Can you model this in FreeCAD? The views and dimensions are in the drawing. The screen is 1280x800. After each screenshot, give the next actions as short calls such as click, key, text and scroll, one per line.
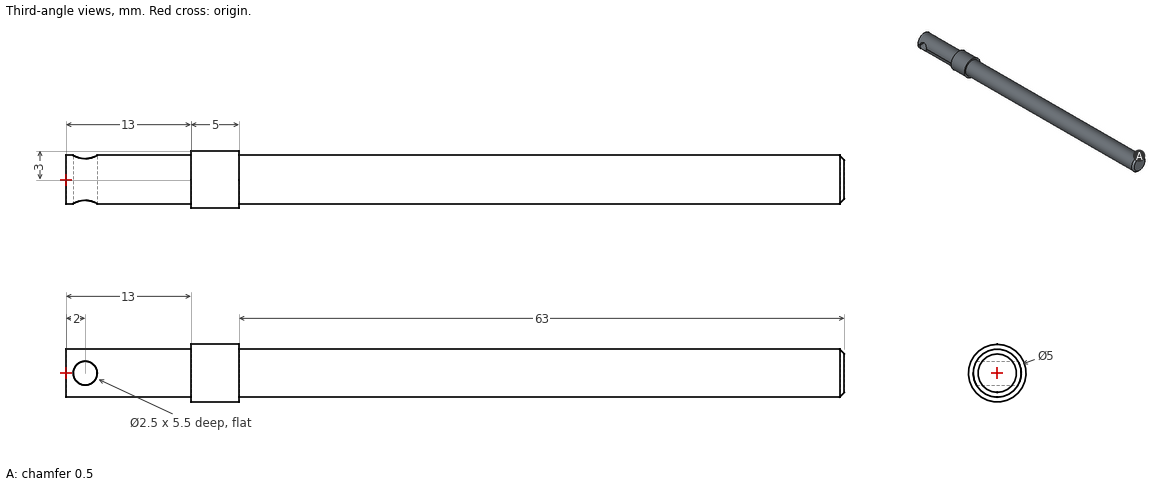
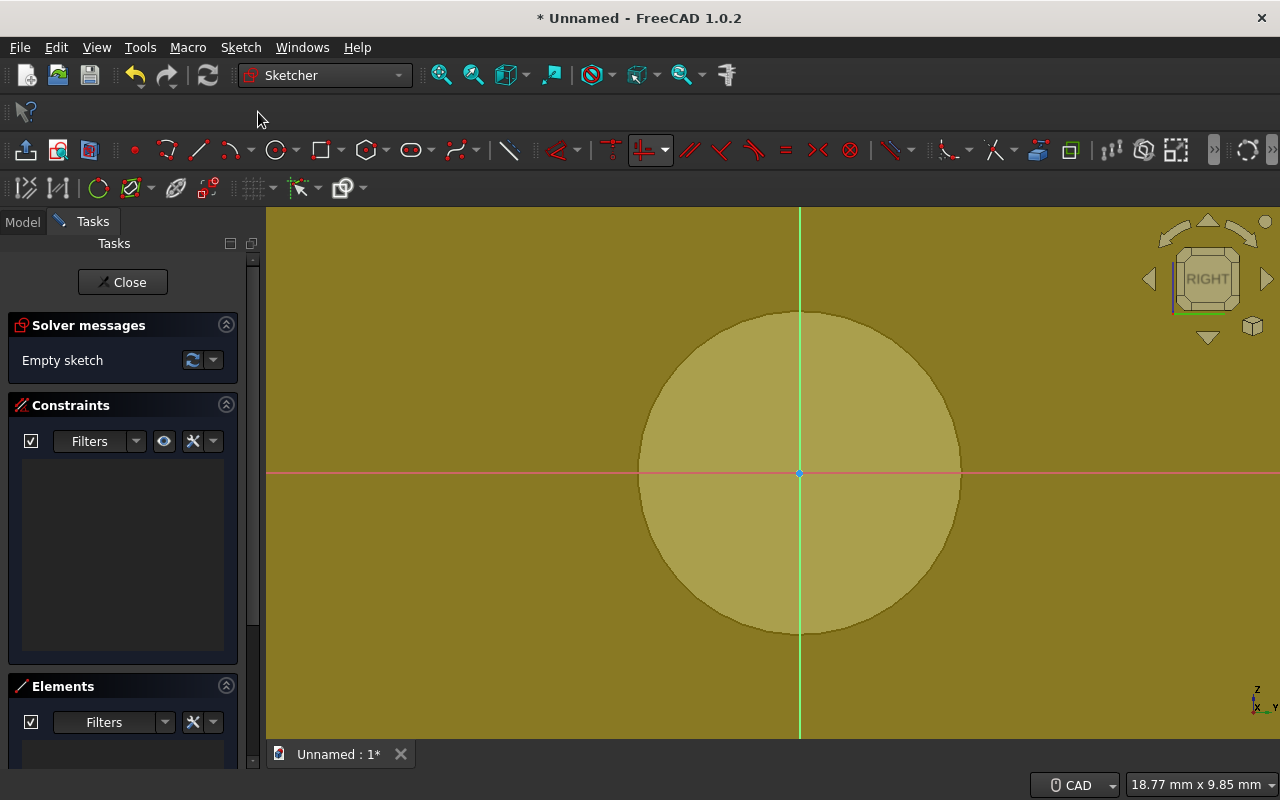
click(276, 150)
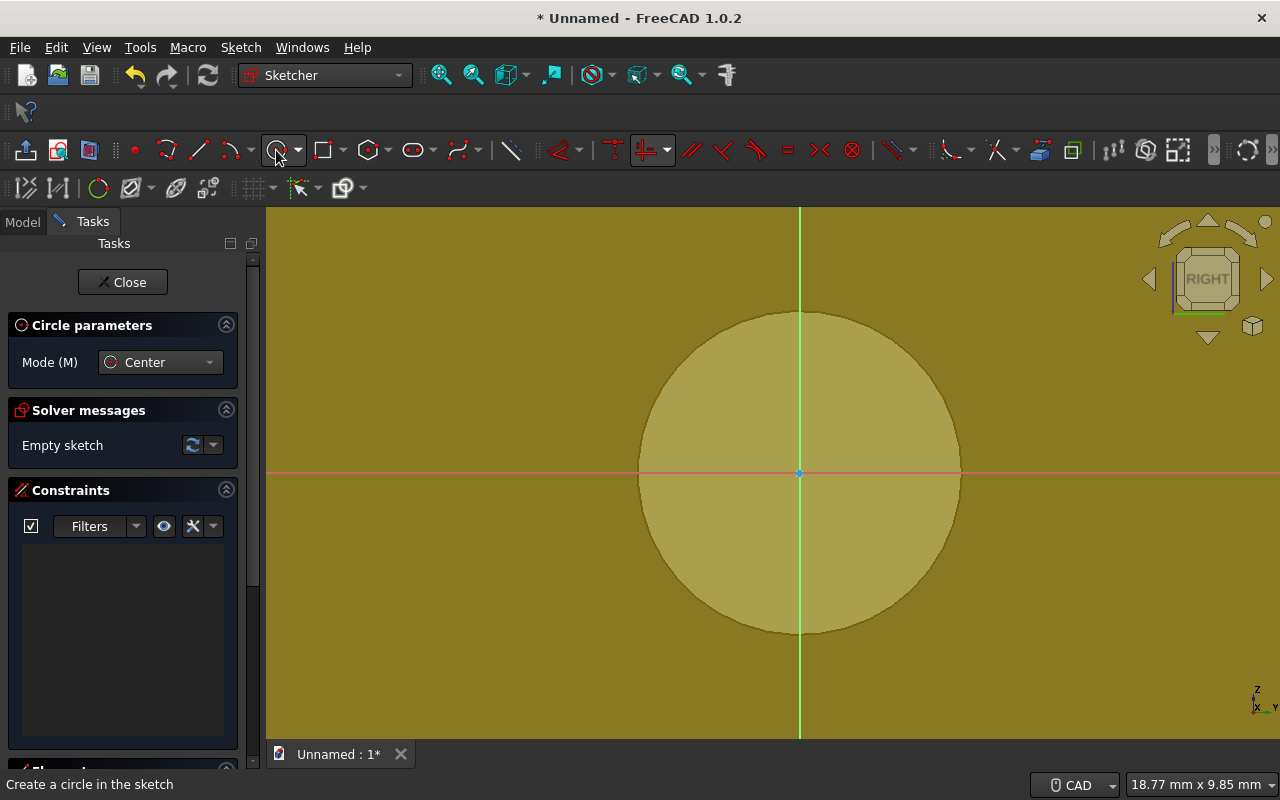
click(800, 473)
move(895, 378)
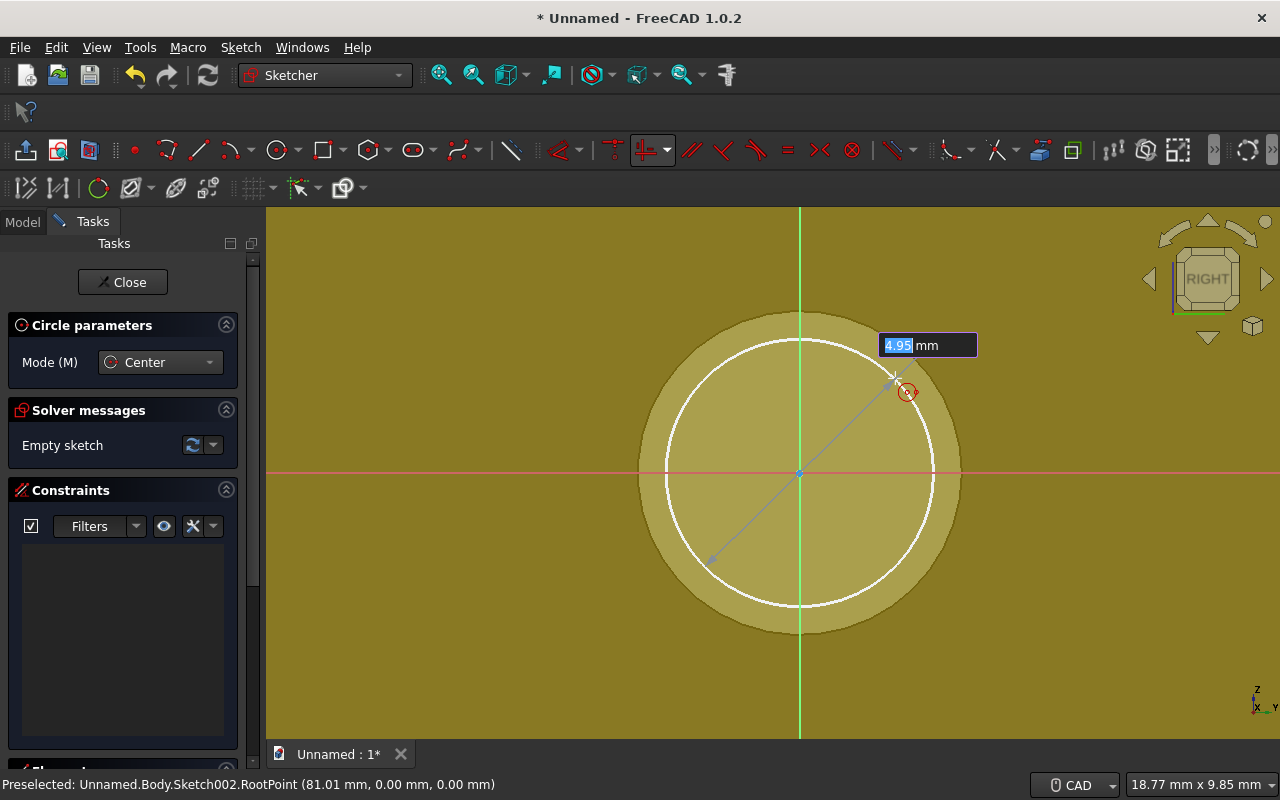
text(5)
key(Return)
key(Escape)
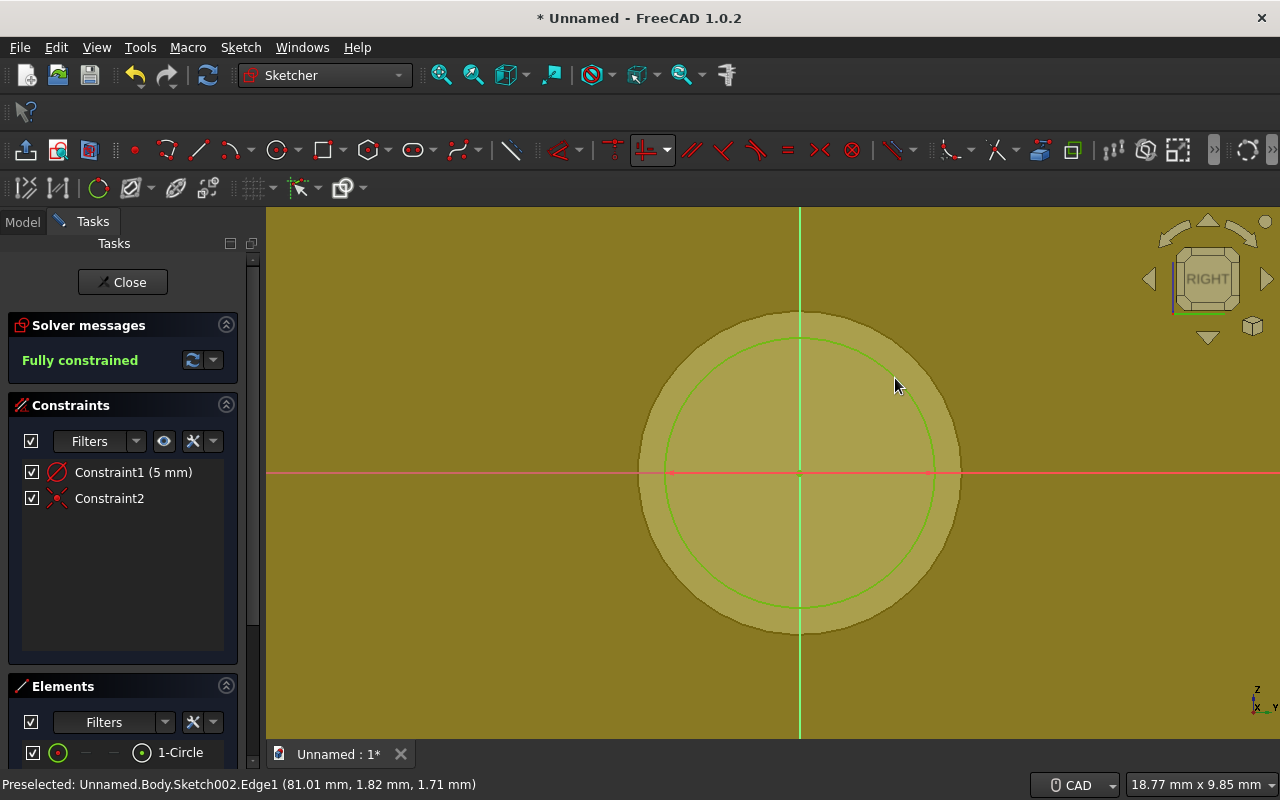
click(123, 282)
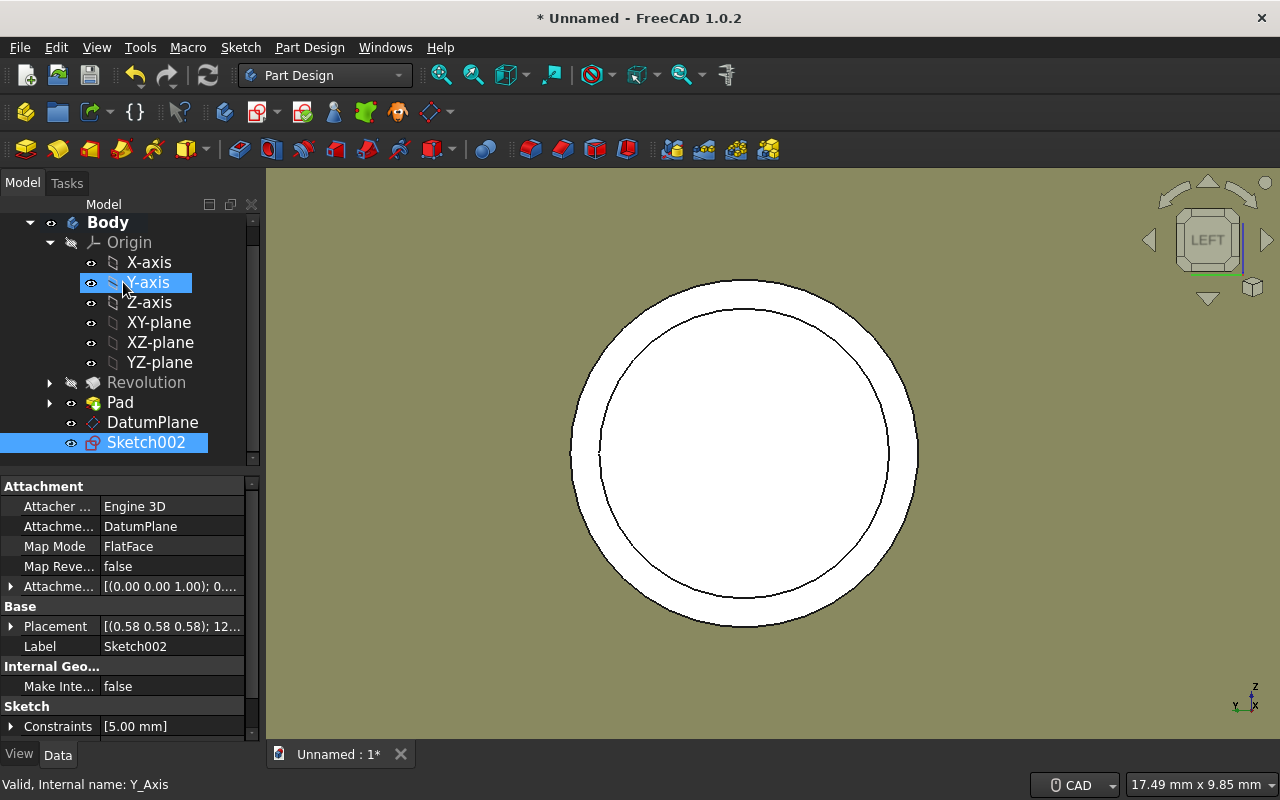
click(26, 150)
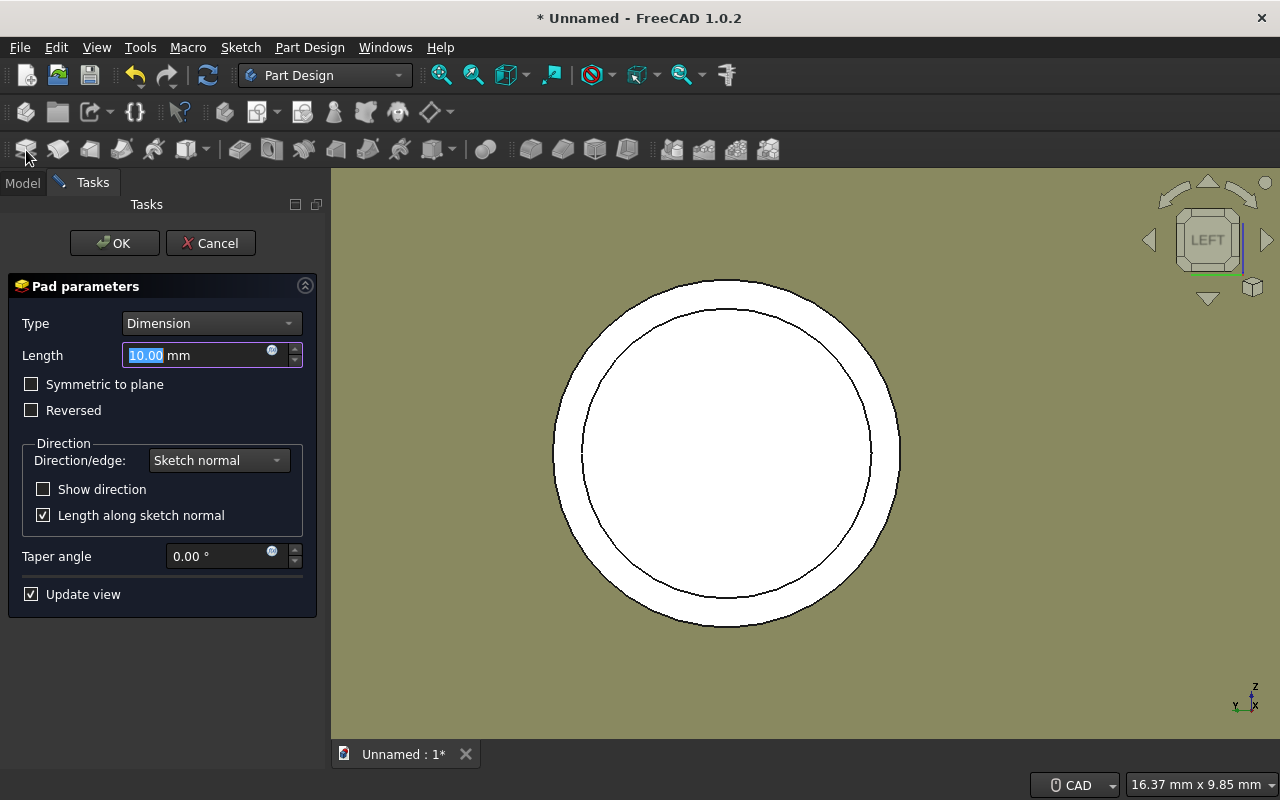
text(63)
key(Tab)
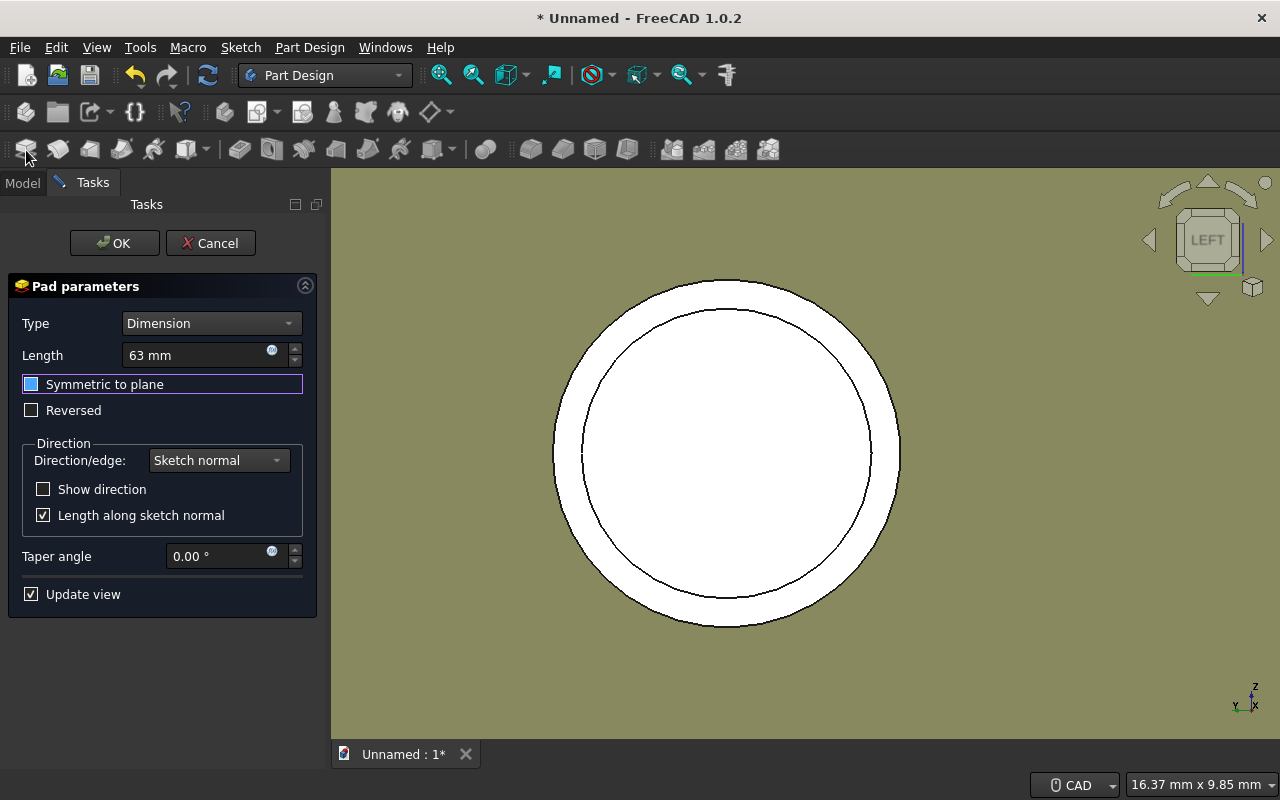
click(30, 410)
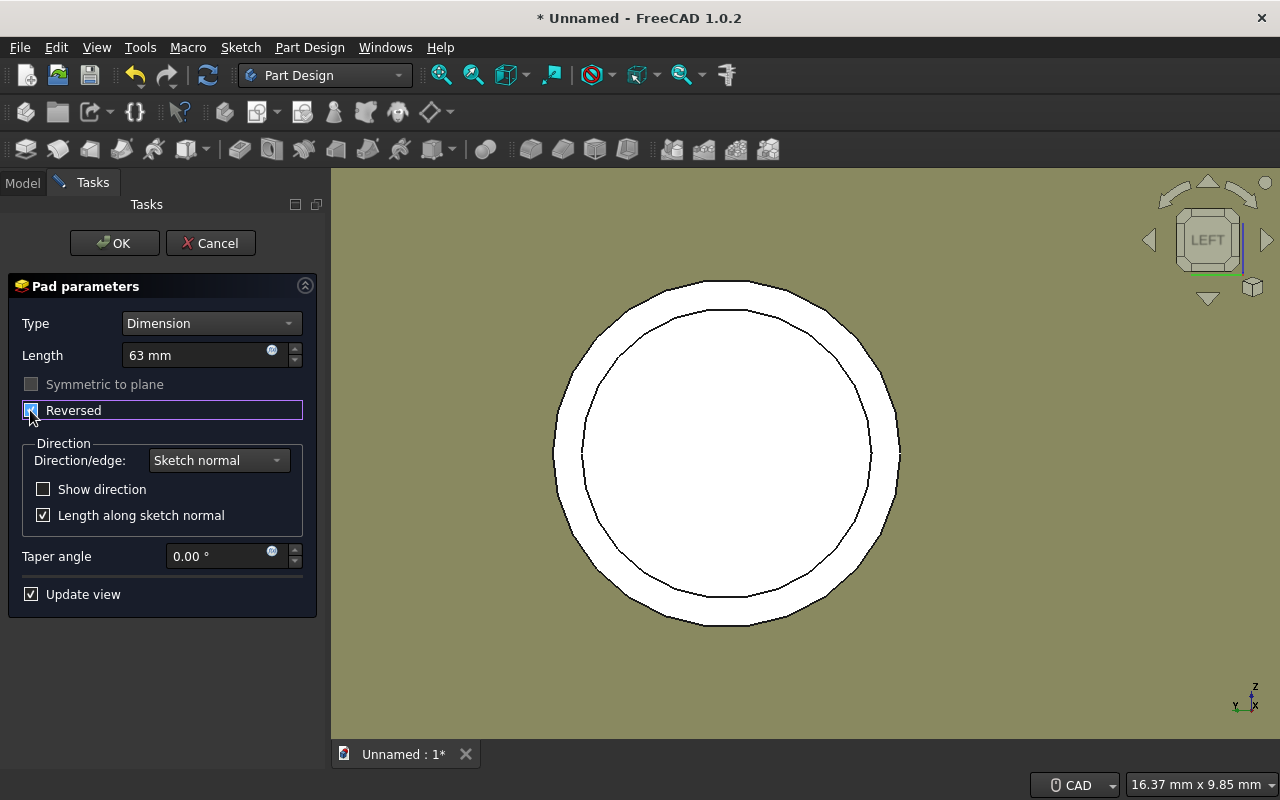
click(115, 243)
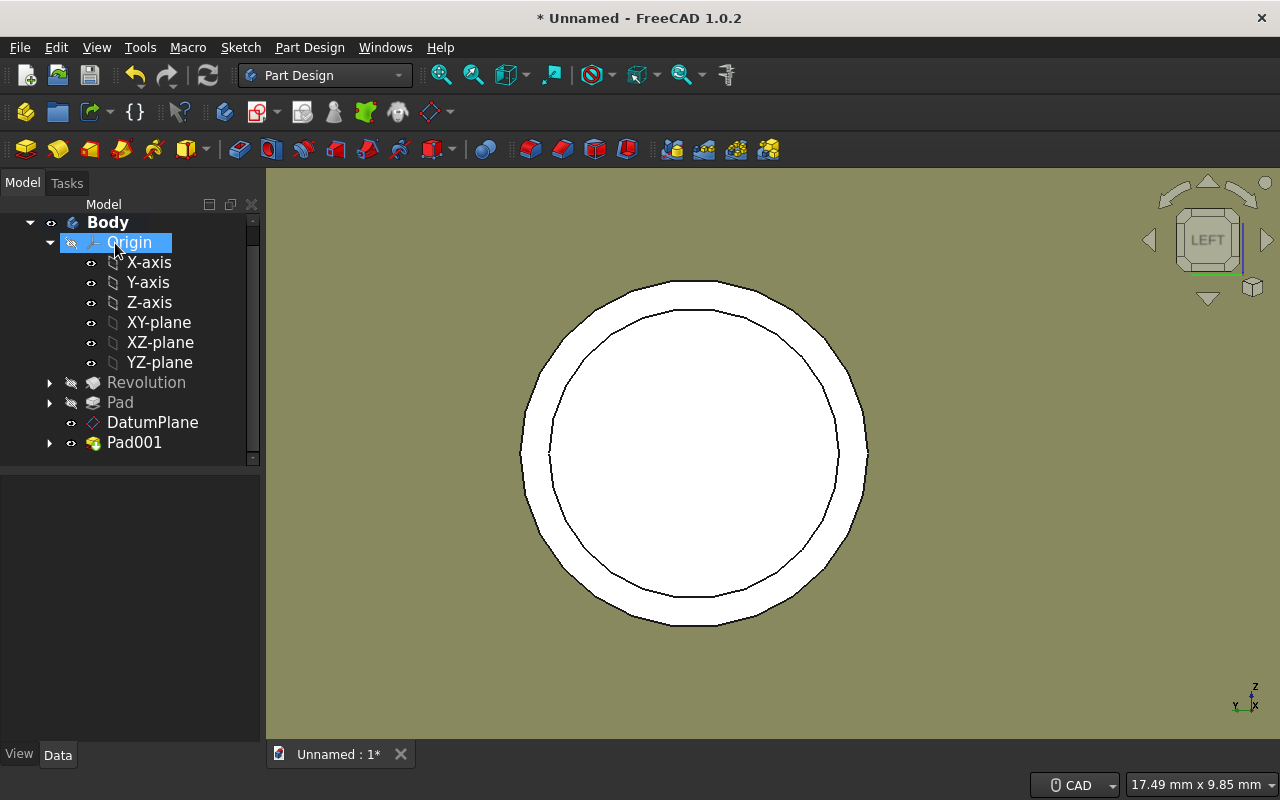
click(116, 423)
key(space)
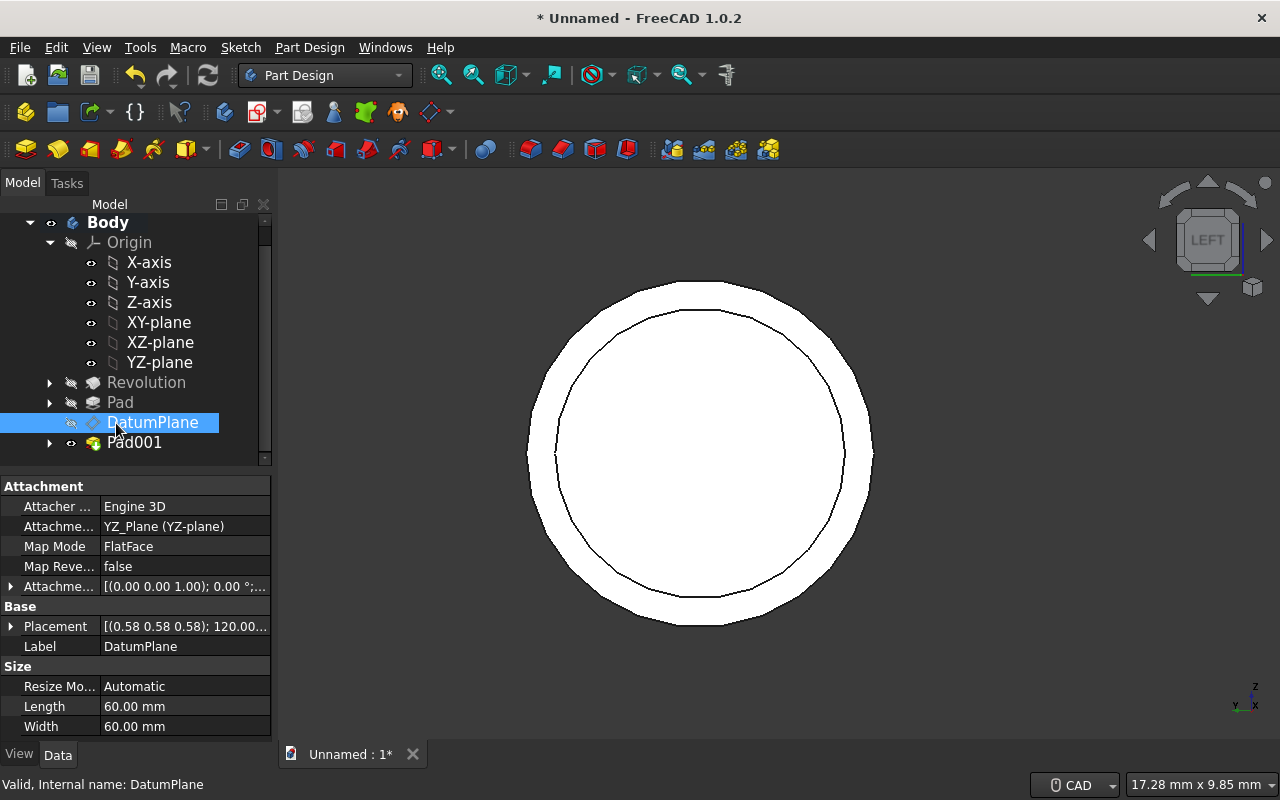
click(136, 343)